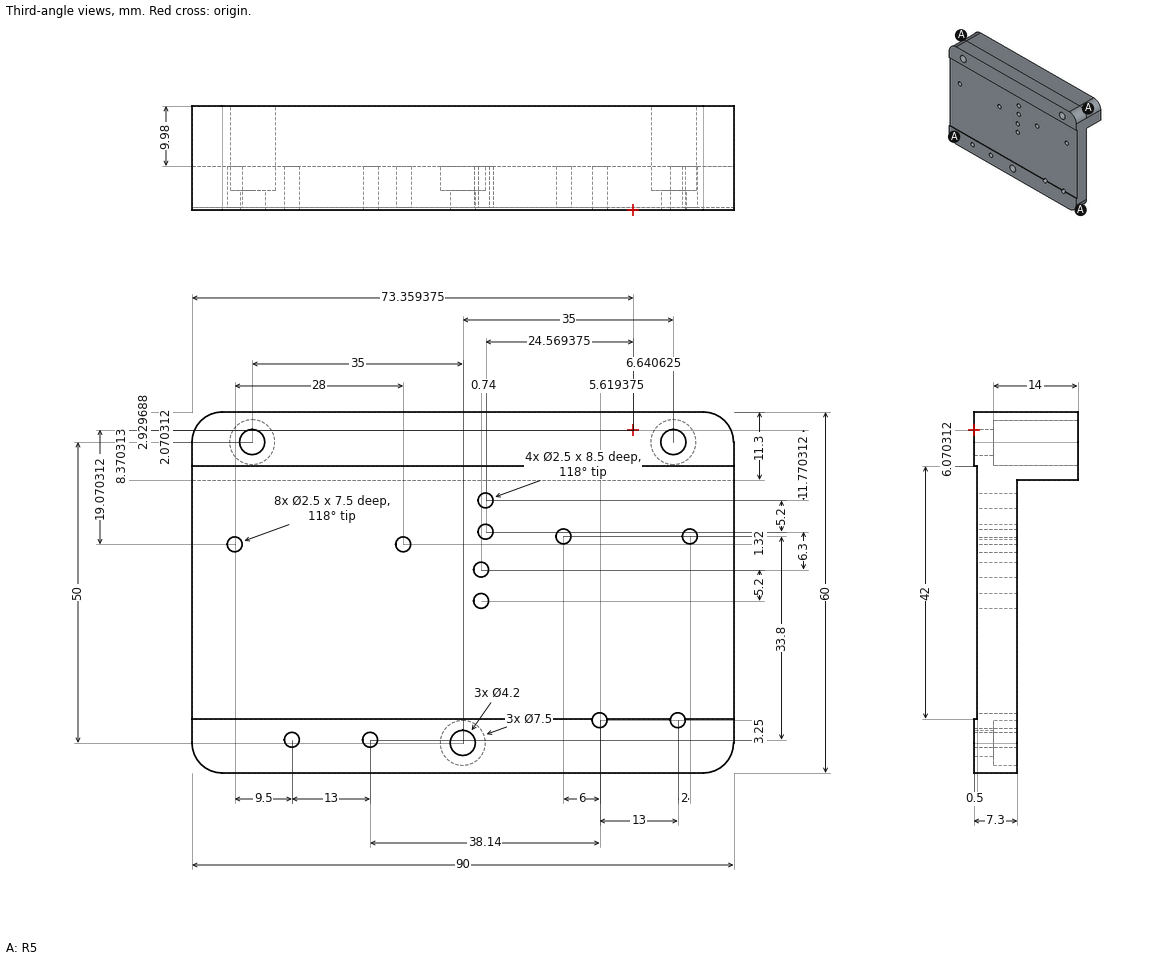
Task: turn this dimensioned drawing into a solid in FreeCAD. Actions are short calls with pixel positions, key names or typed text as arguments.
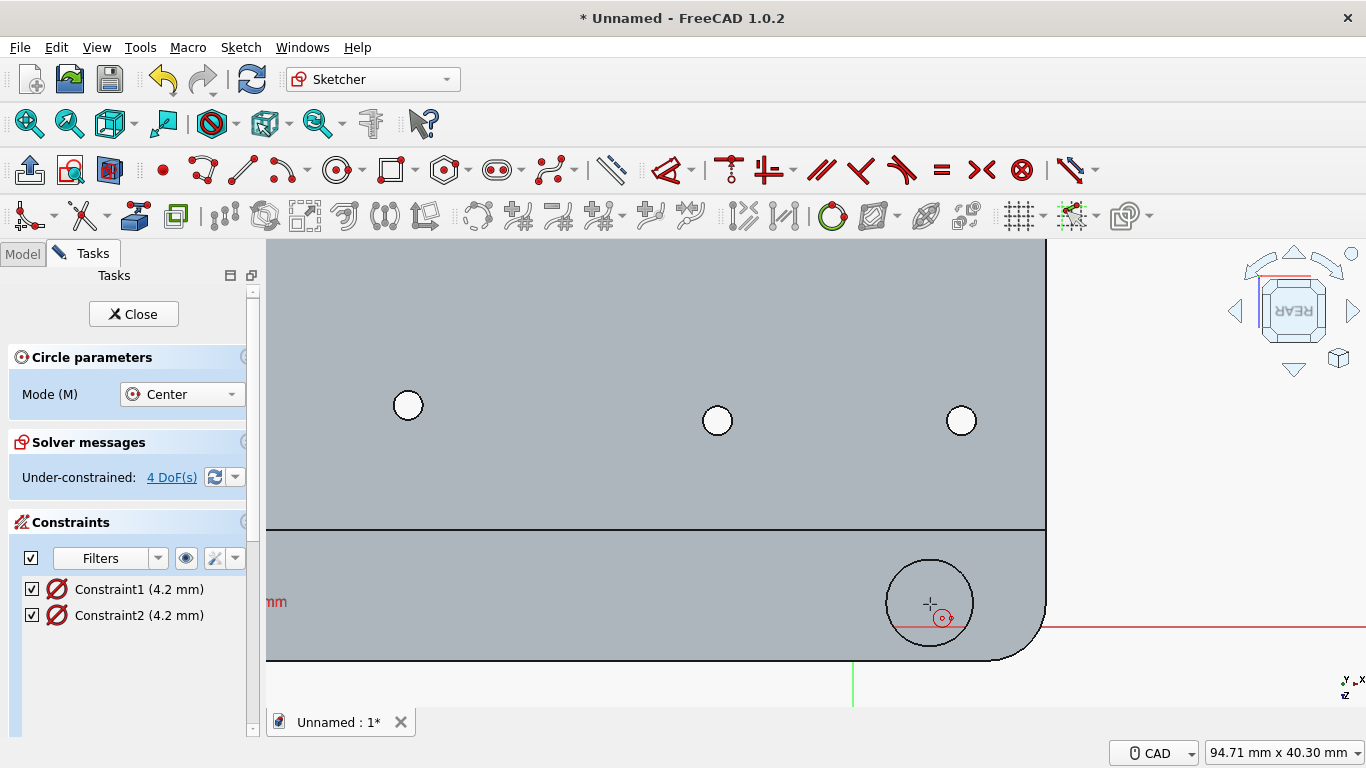
click(930, 603)
move(947, 586)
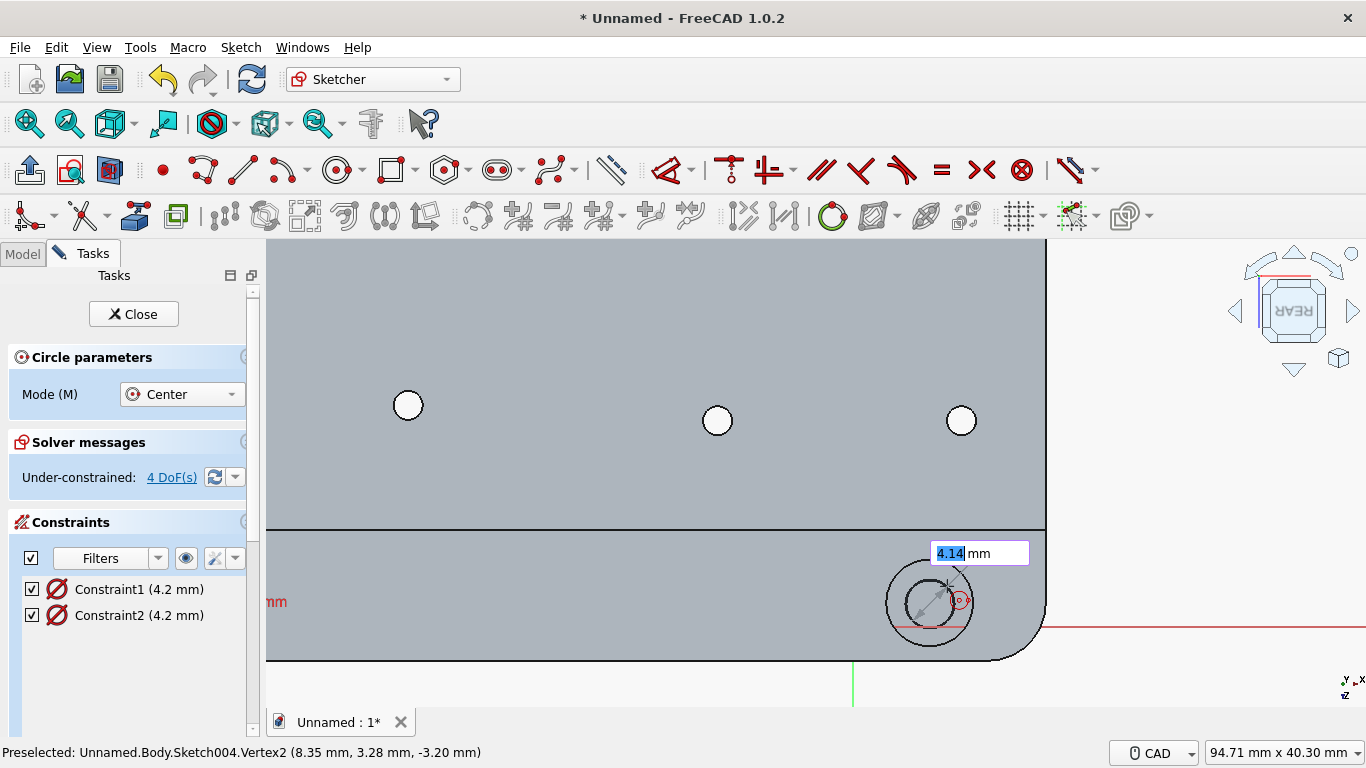
text(4.2)
key(Return)
key(Escape)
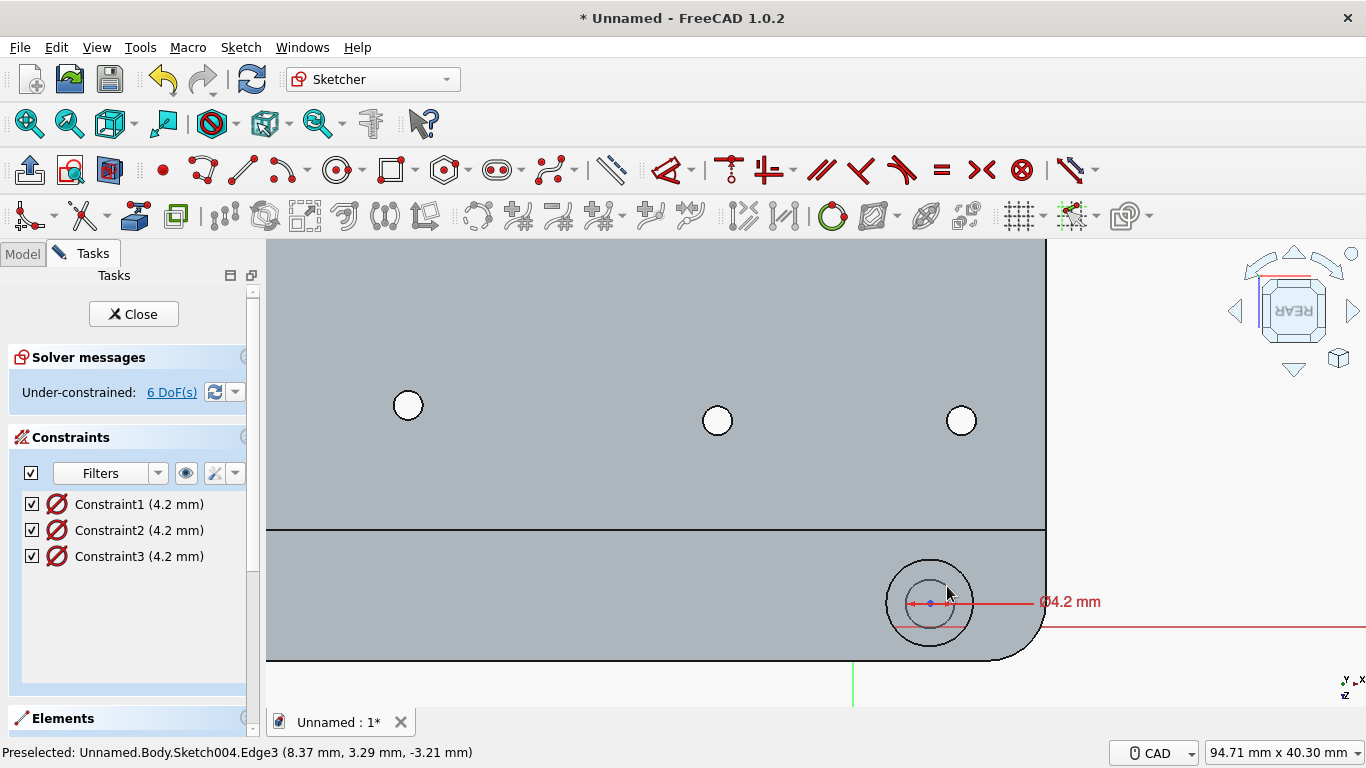
click(666, 170)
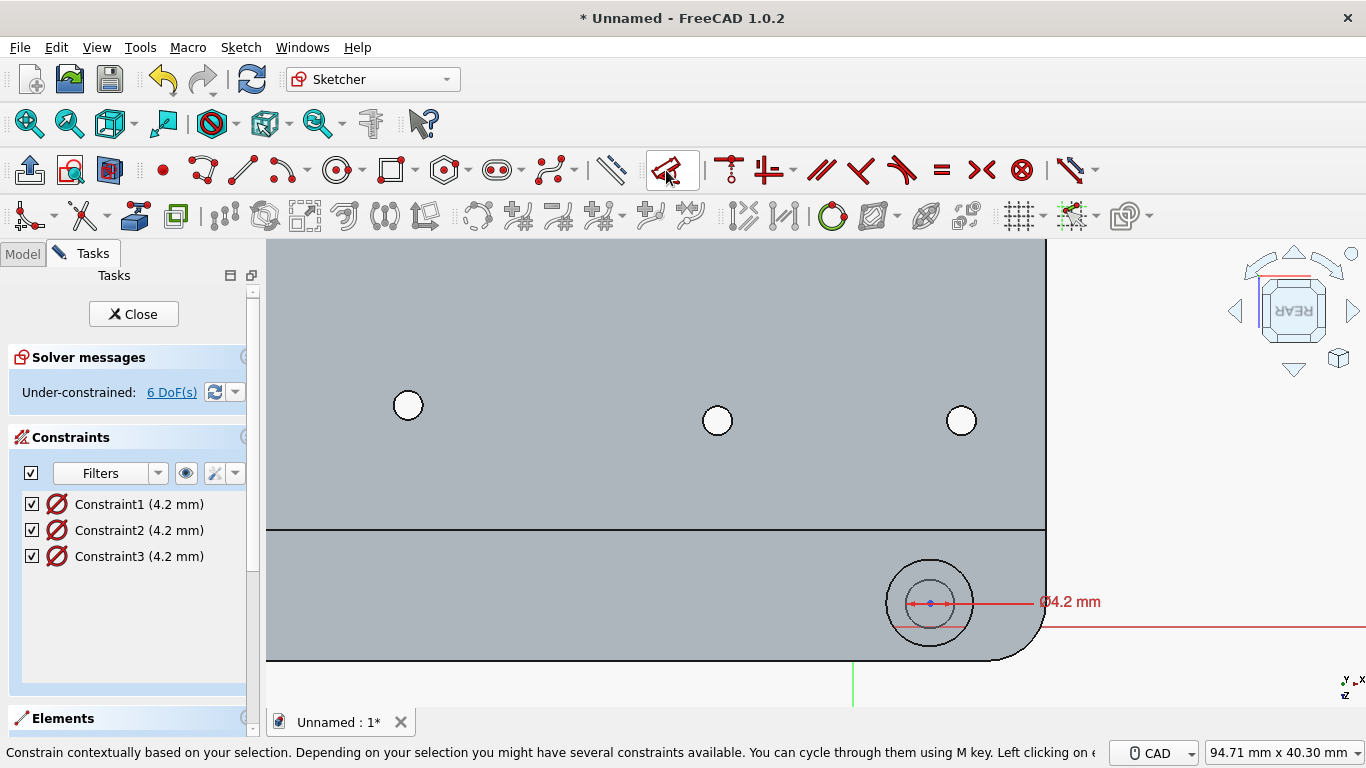
scroll(931, 604, down, 4)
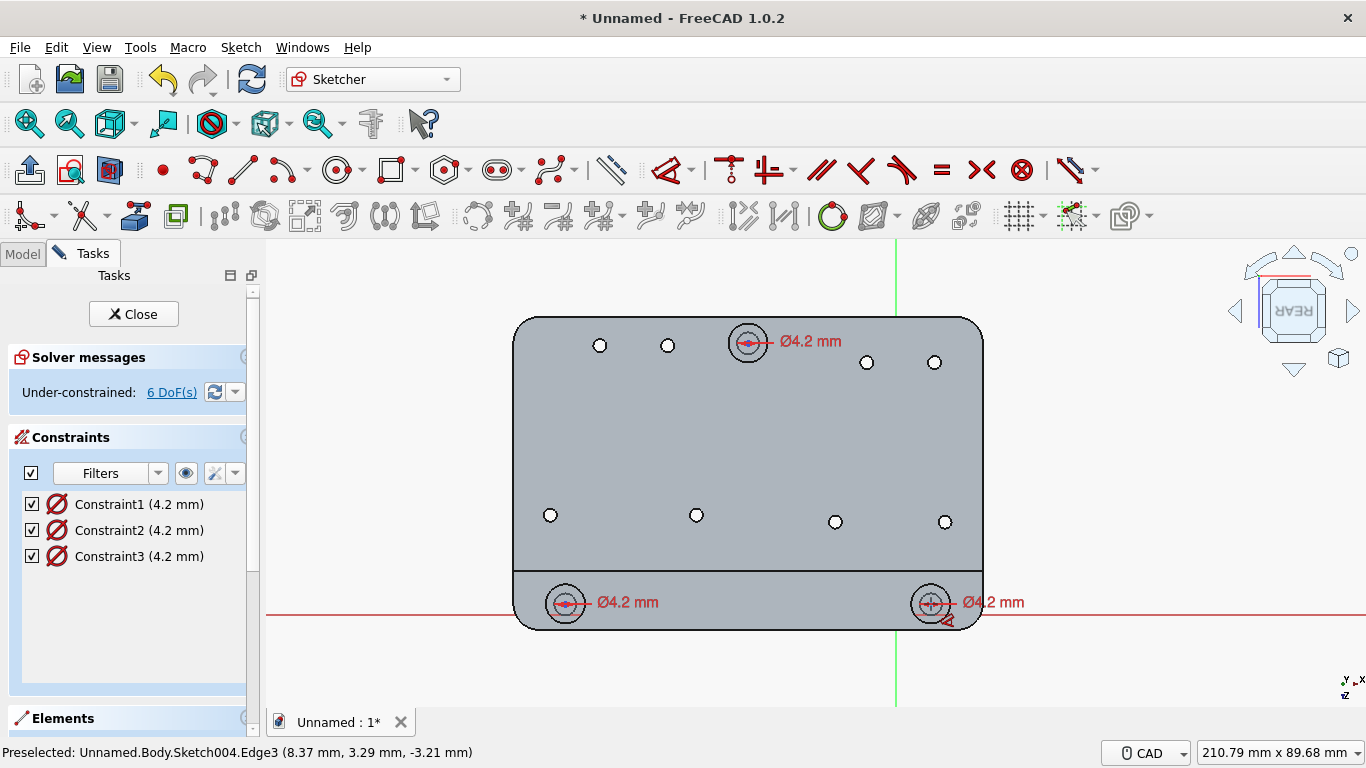
click(748, 343)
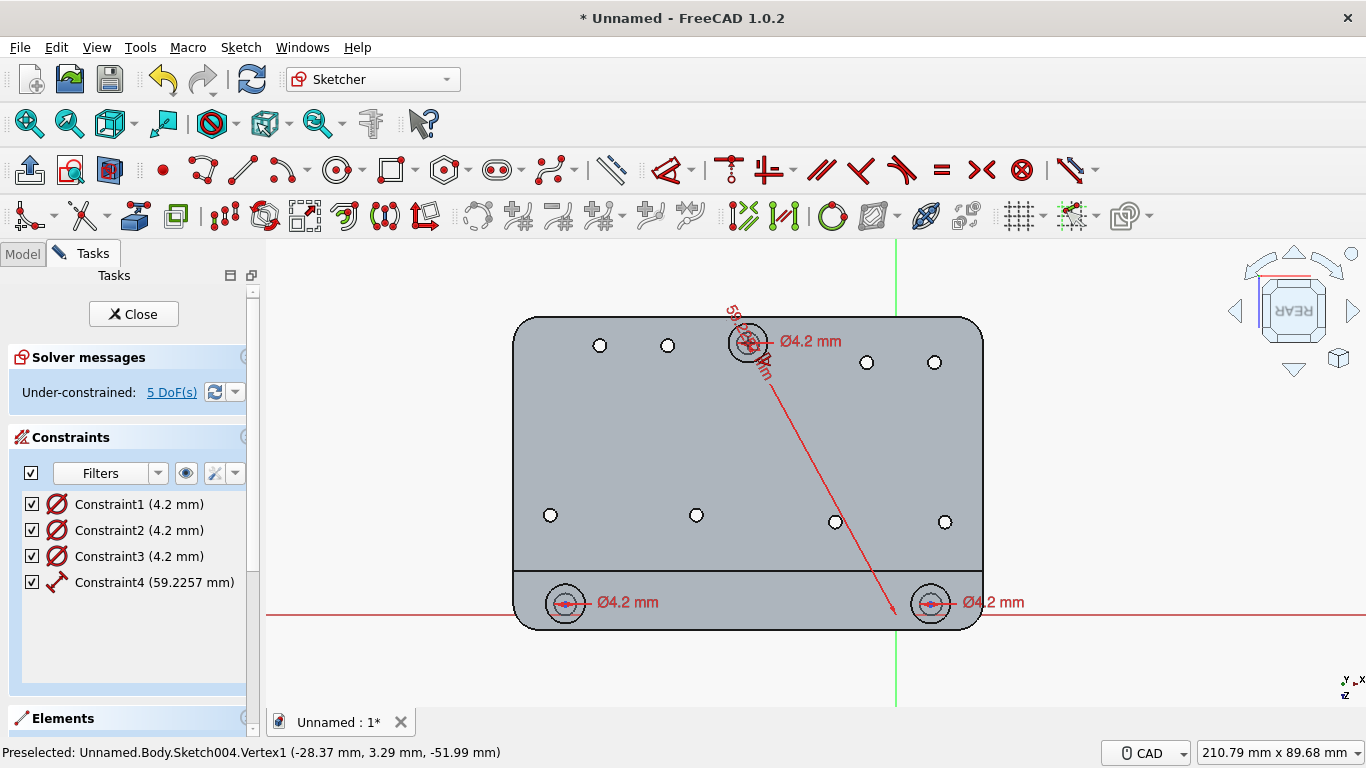
click(565, 604)
click(657, 638)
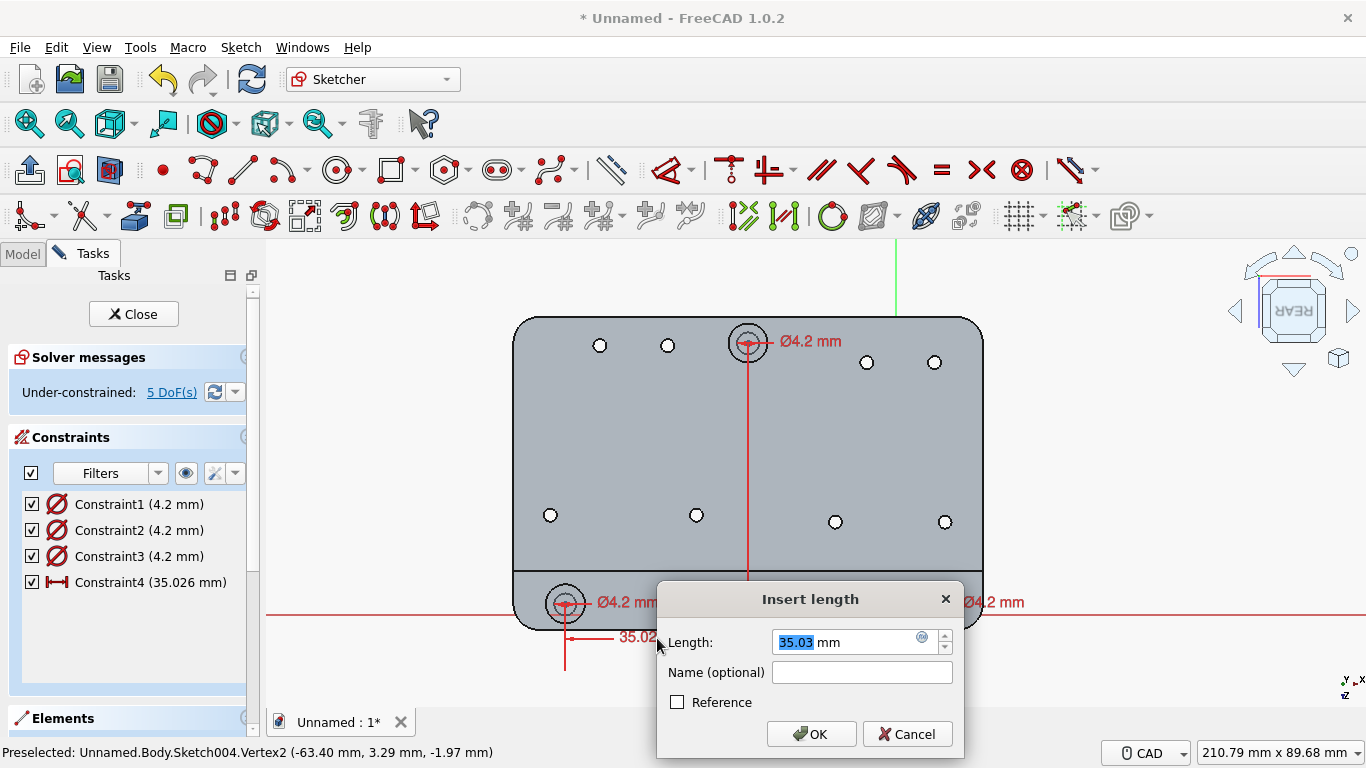
text(35)
key(Return)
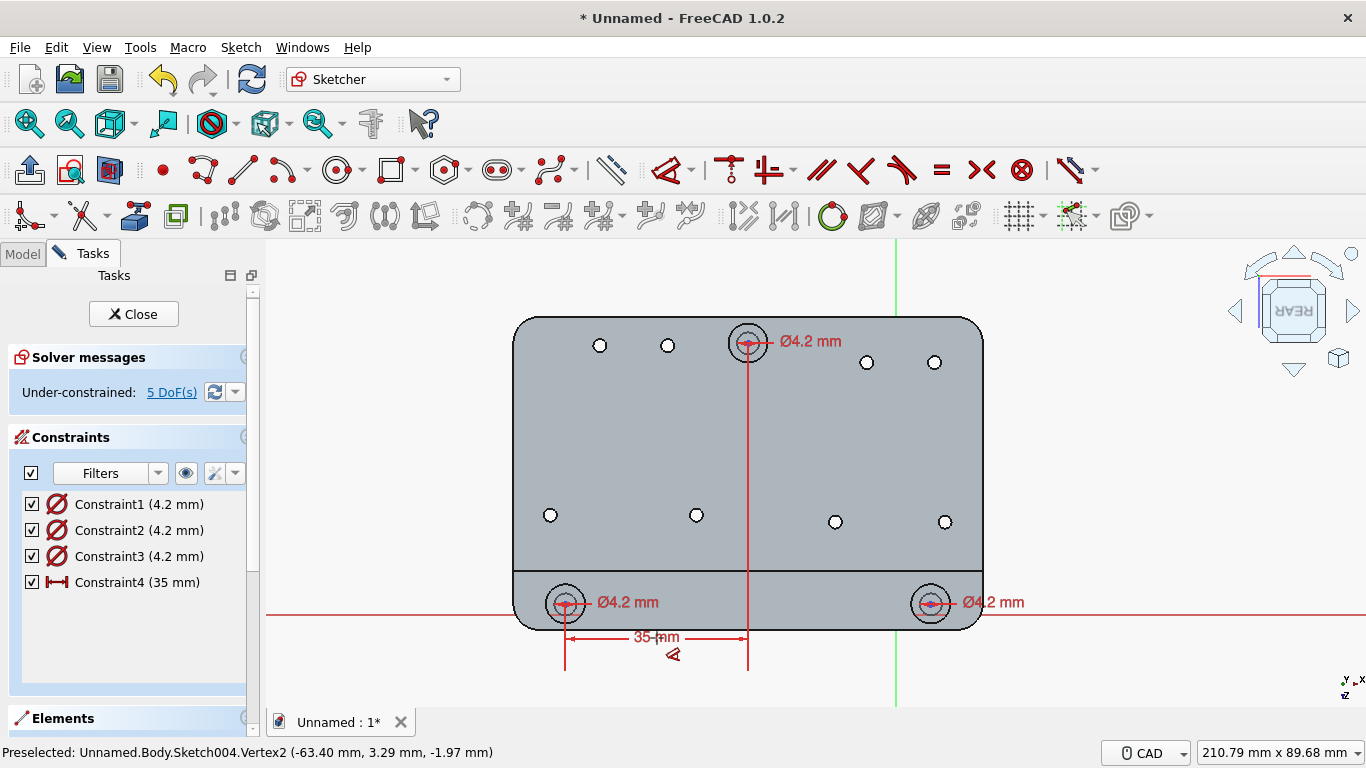
click(748, 343)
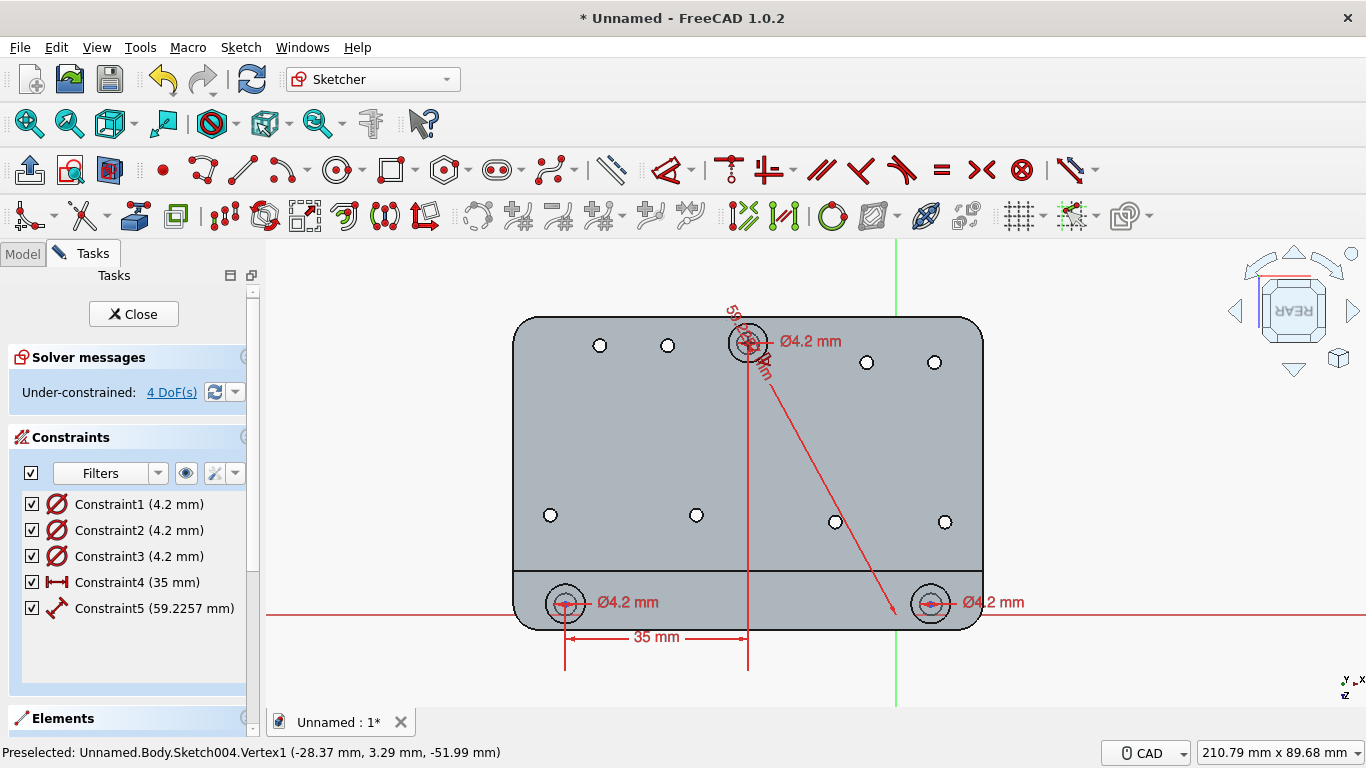
click(565, 604)
click(531, 474)